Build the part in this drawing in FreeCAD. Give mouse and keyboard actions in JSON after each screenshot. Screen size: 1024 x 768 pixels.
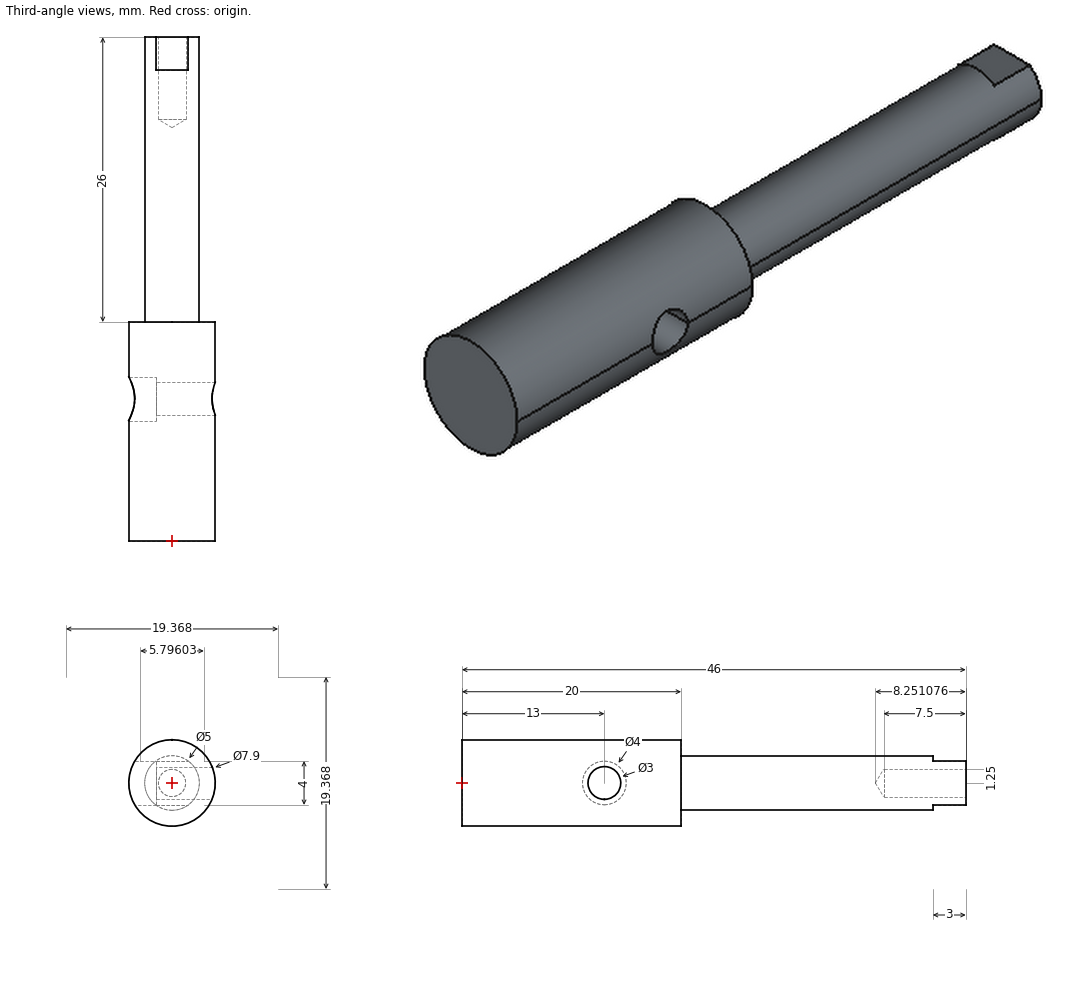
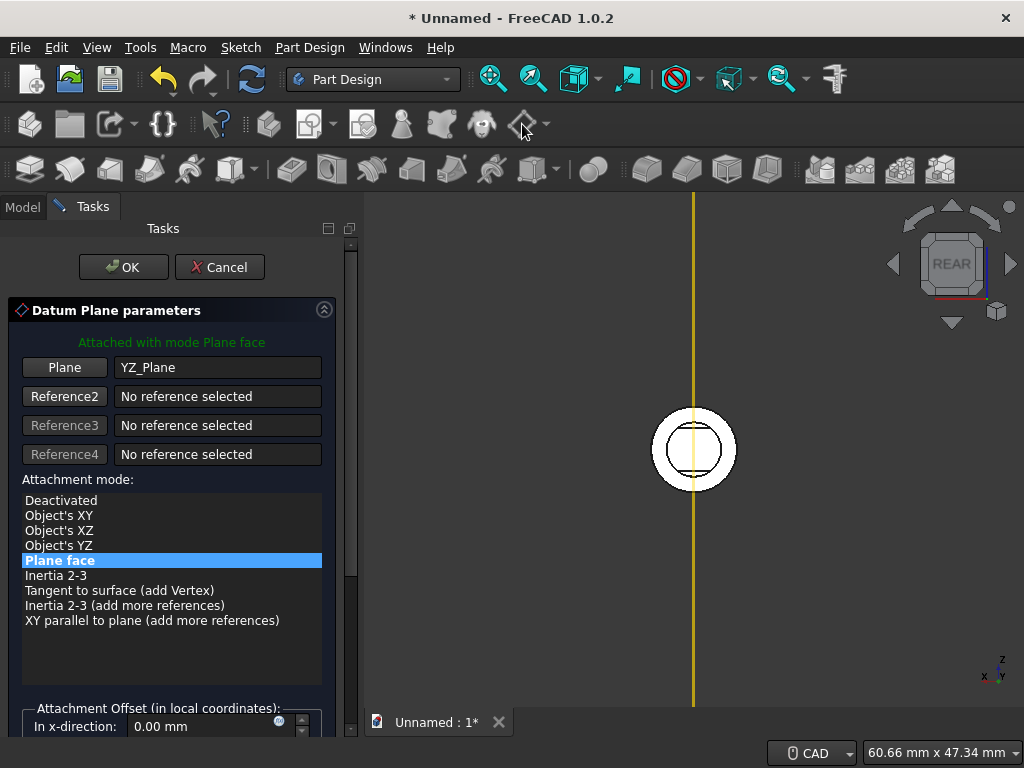
{"action": "scroll", "coordinate": [351, 487], "scroll_direction": "down", "scroll_amount": 3}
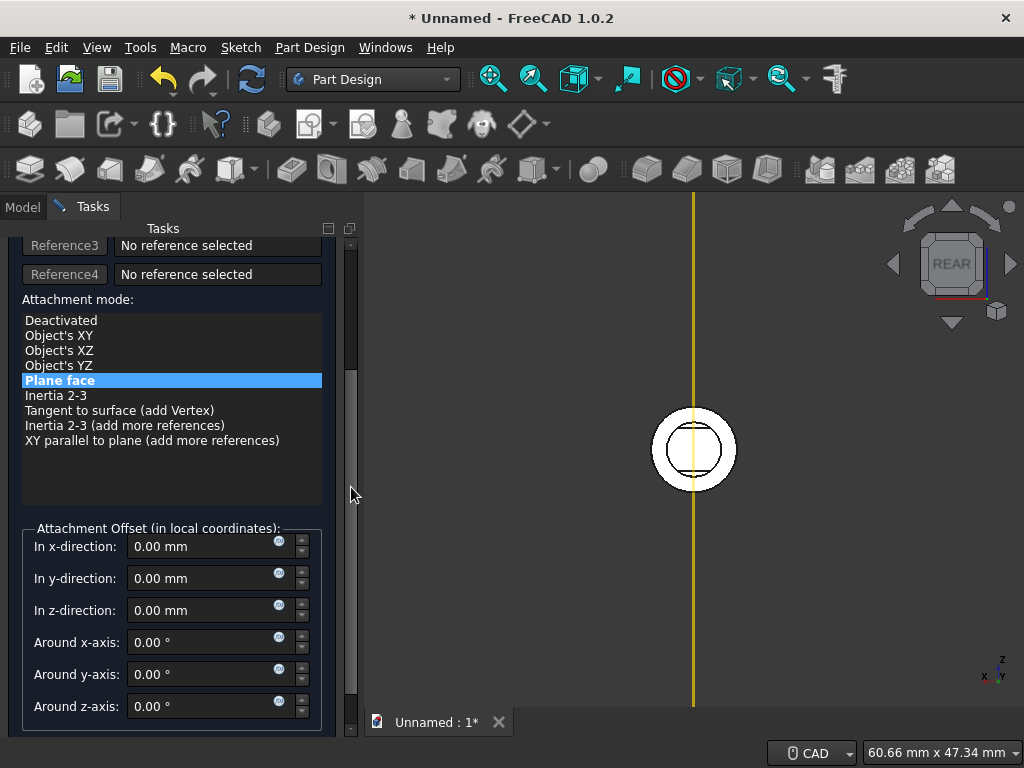
{"action": "triple_click", "coordinate": [210, 610]}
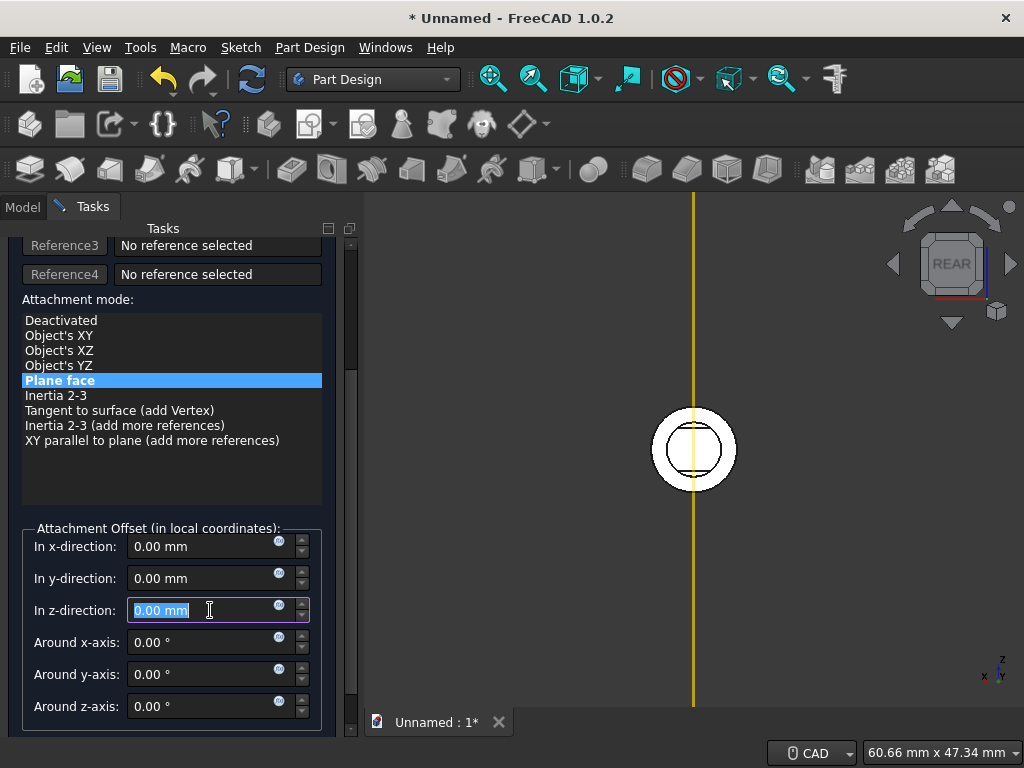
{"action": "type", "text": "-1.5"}
{"action": "key", "text": "Tab"}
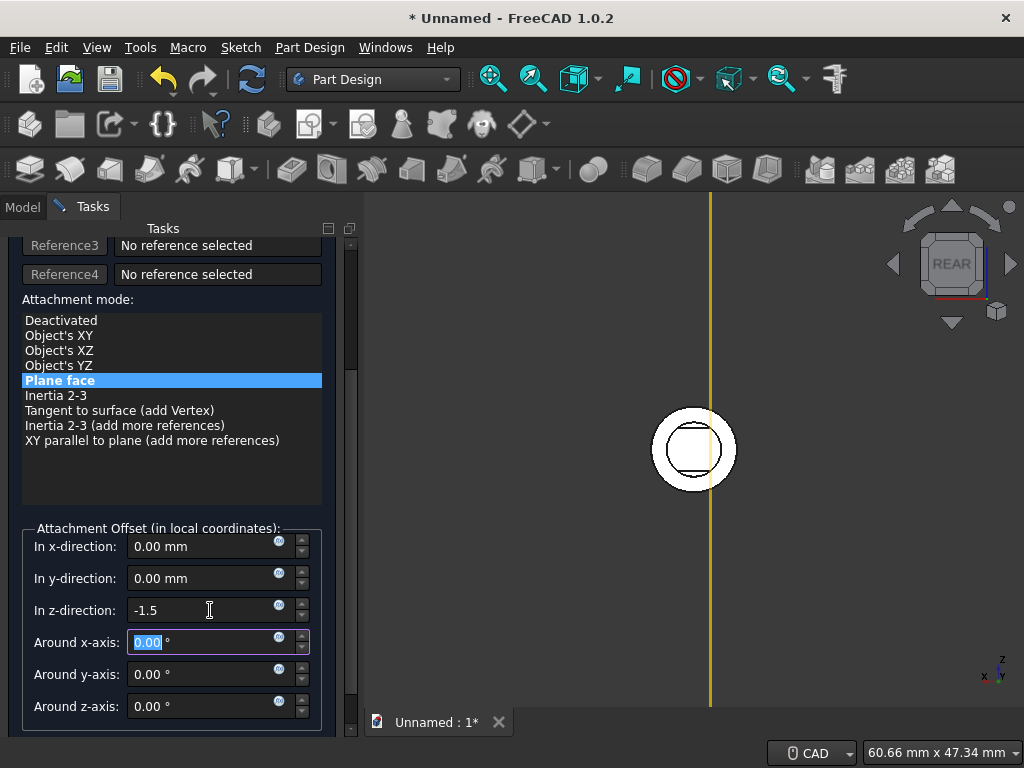
{"action": "scroll", "coordinate": [351, 487], "scroll_direction": "up", "scroll_amount": 4}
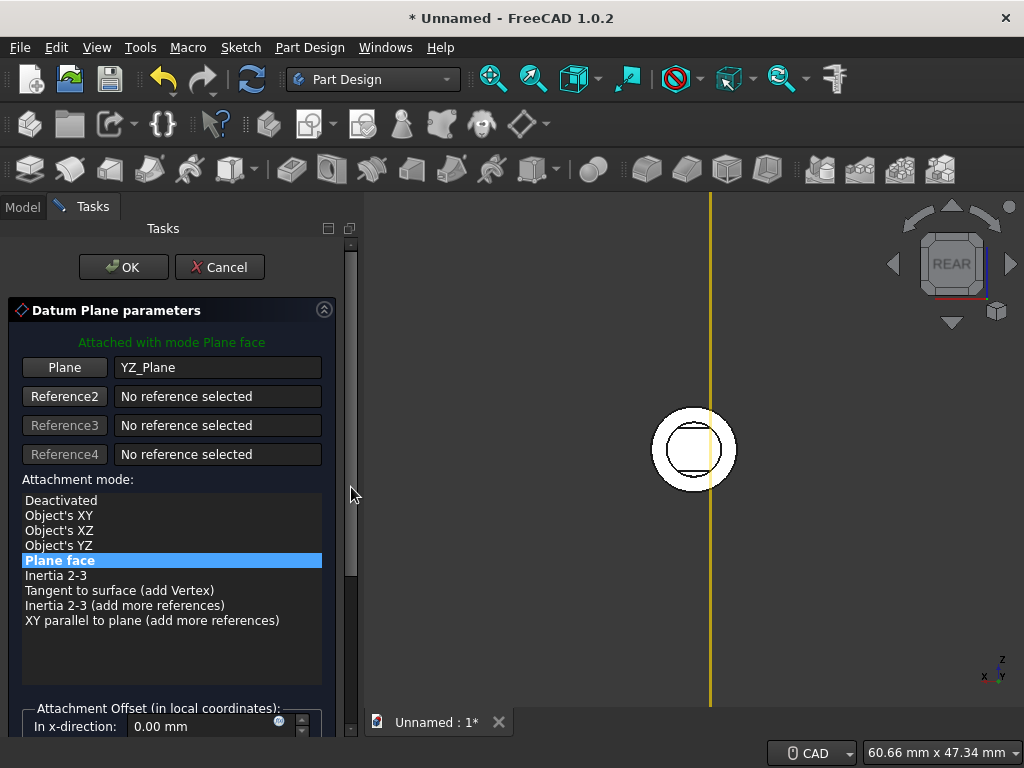
{"action": "left_click", "coordinate": [124, 267]}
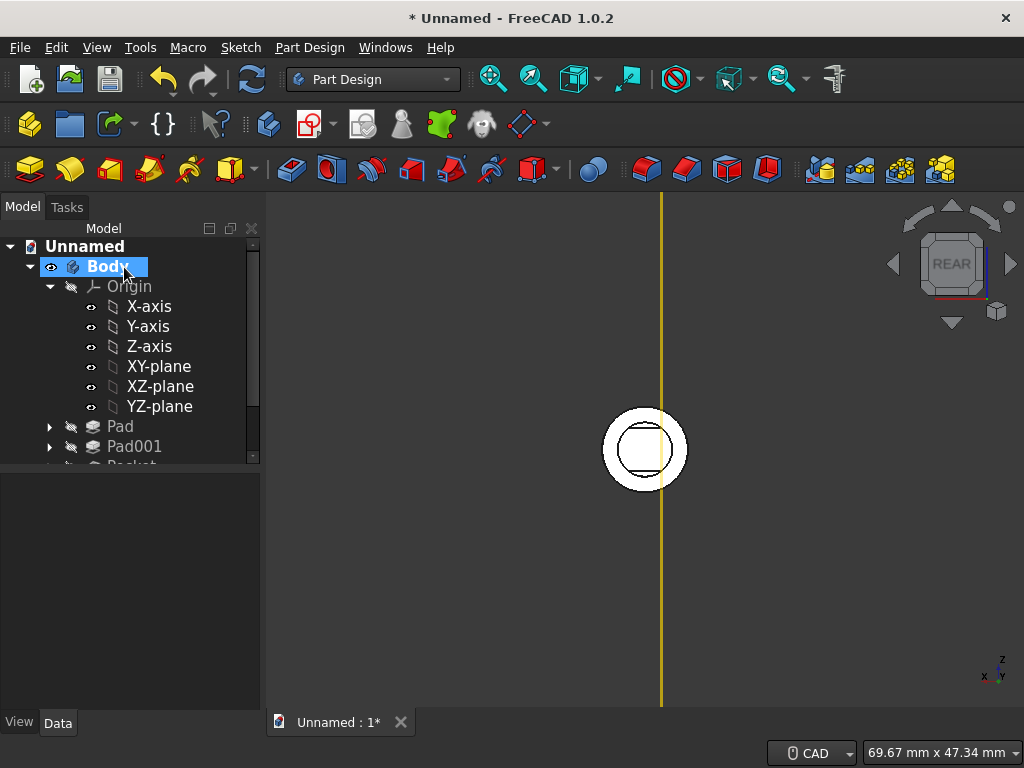
{"action": "scroll", "coordinate": [100, 342], "scroll_direction": "down", "scroll_amount": 3}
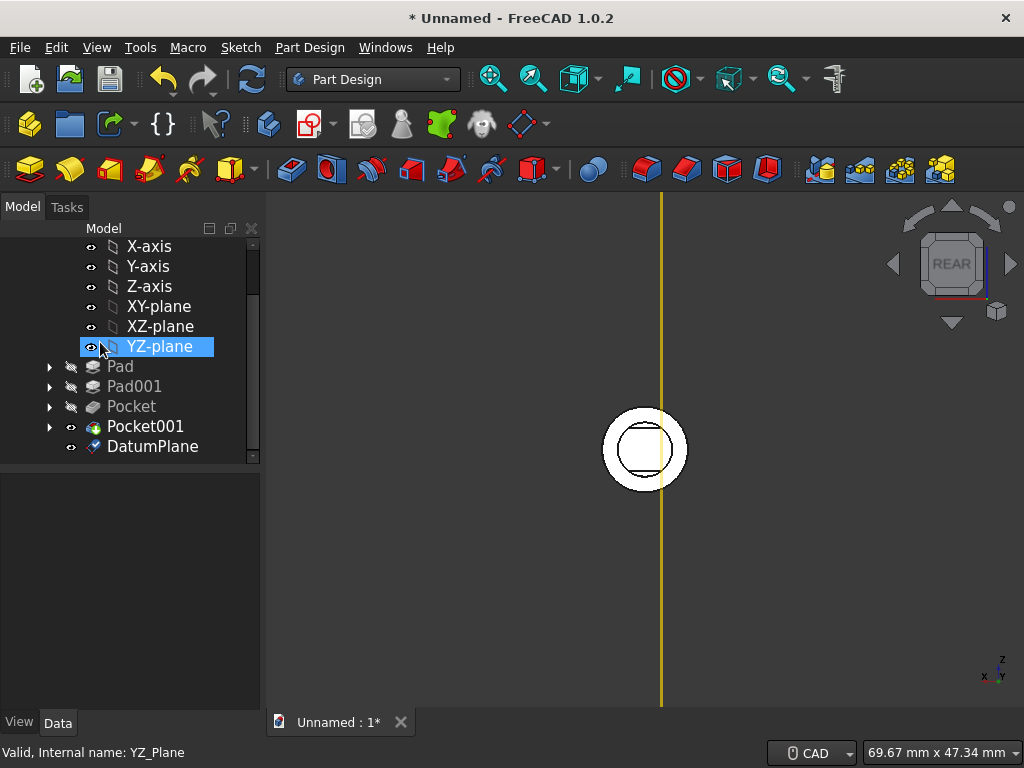
{"action": "left_click", "coordinate": [116, 447]}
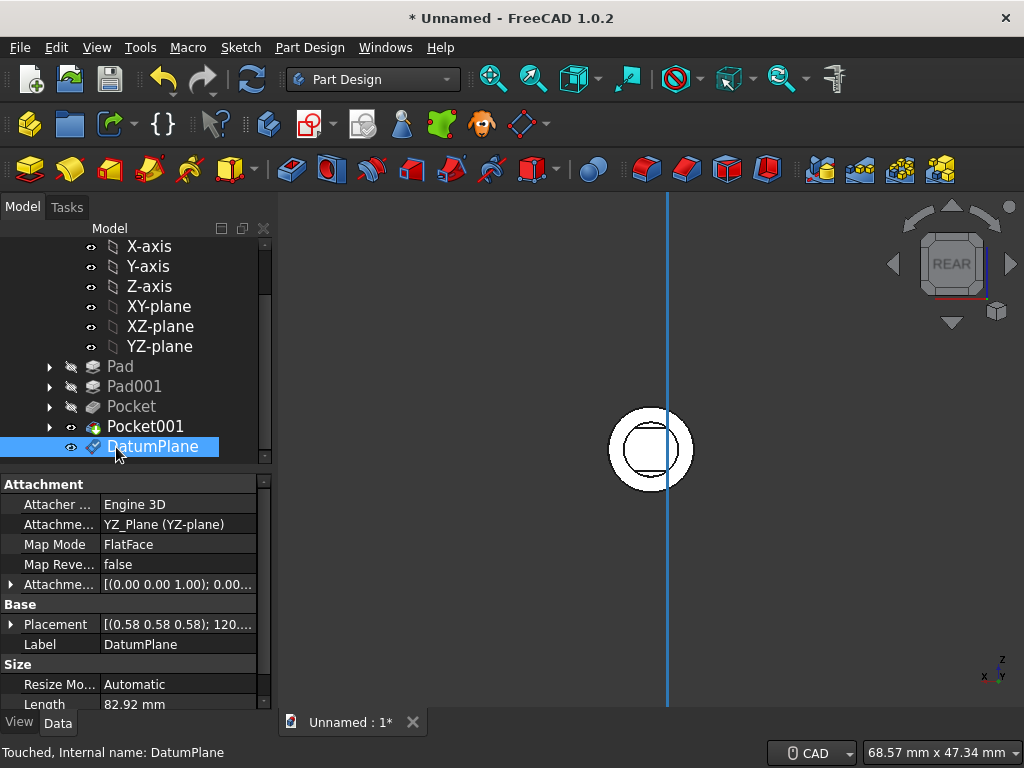
{"action": "left_click", "coordinate": [310, 124]}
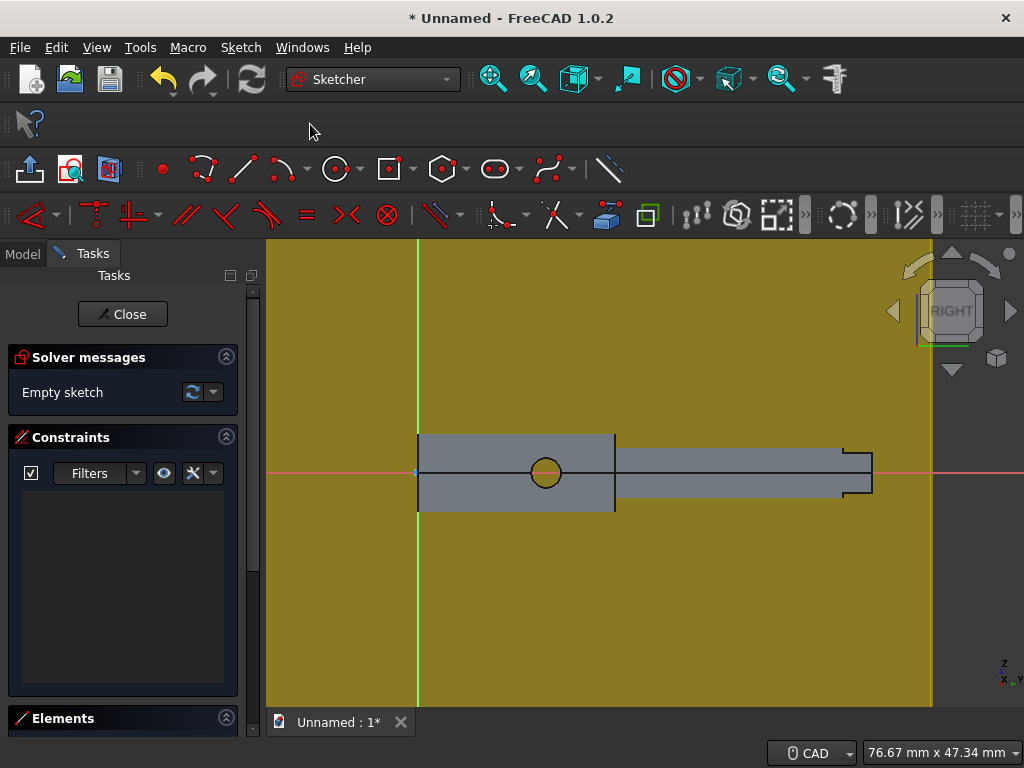
{"action": "left_click", "coordinate": [110, 170]}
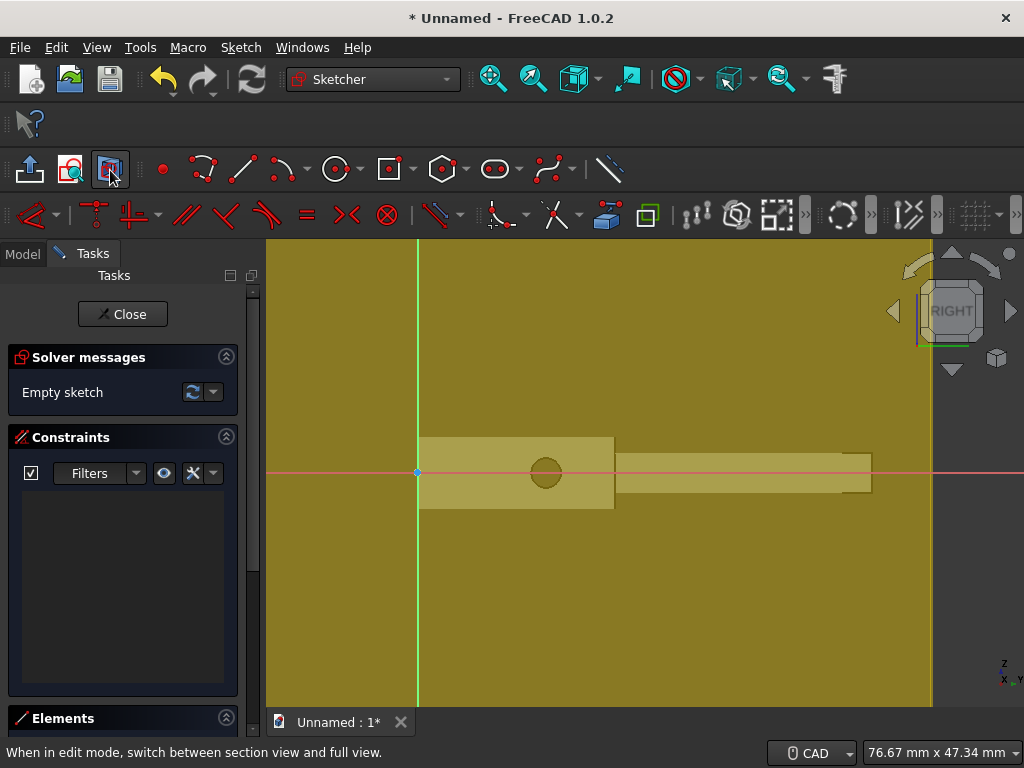
{"action": "scroll", "coordinate": [541, 473], "scroll_direction": "up", "scroll_amount": 10}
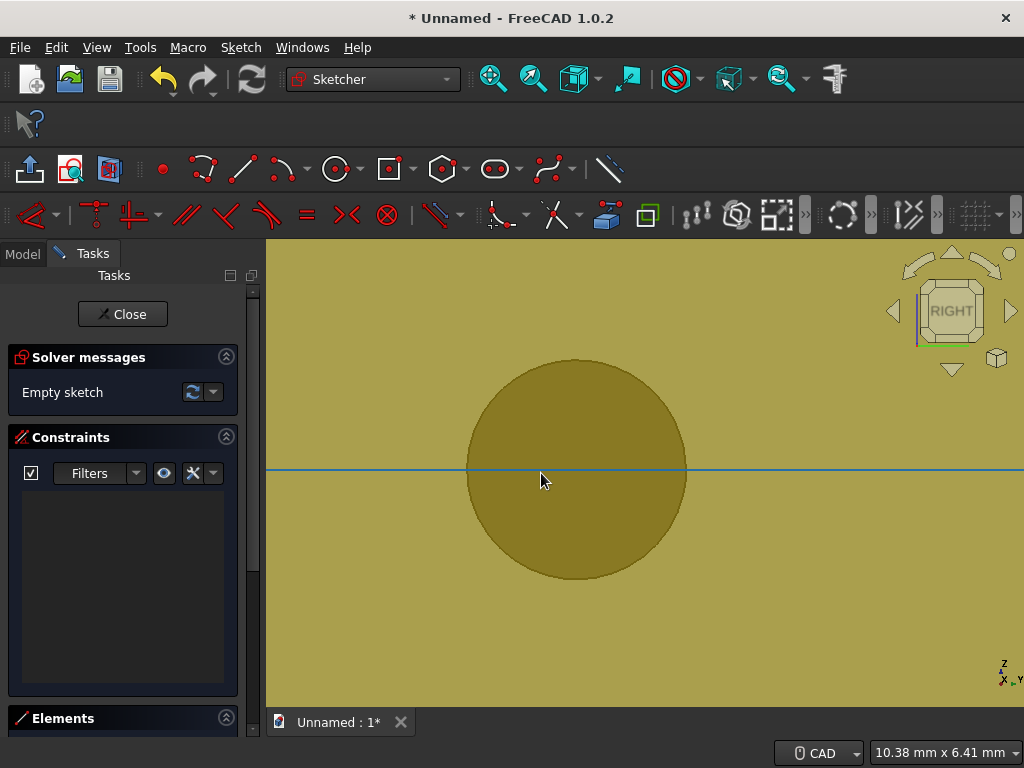
{"action": "left_click", "coordinate": [336, 170]}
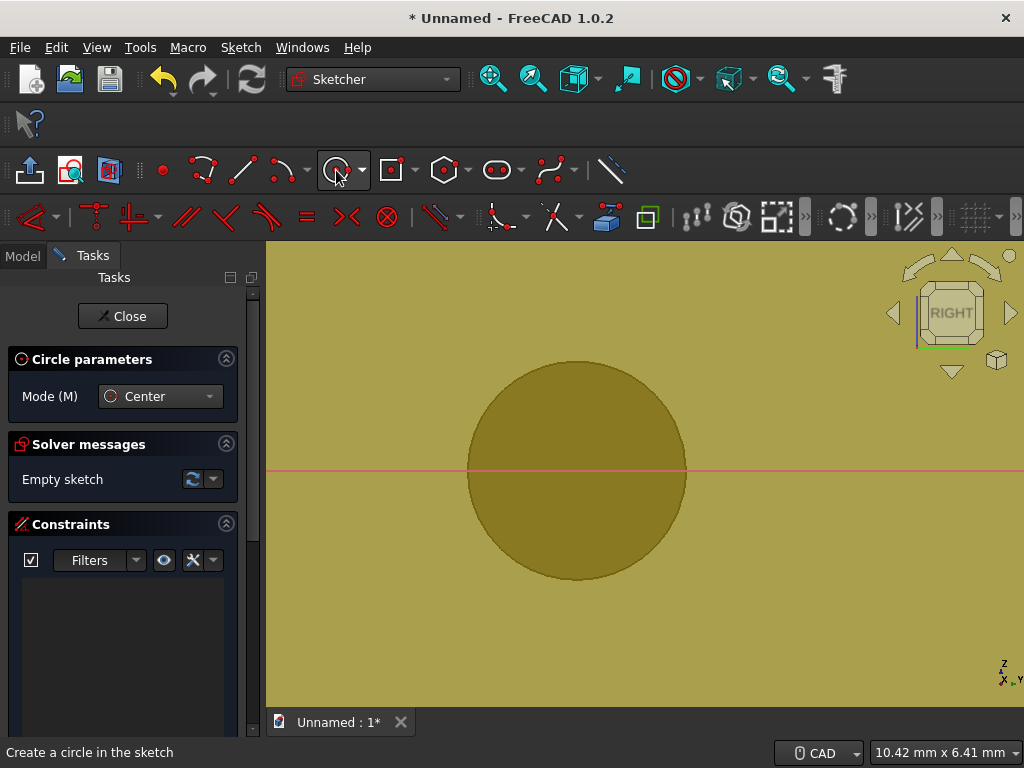
{"action": "left_click", "coordinate": [577, 471]}
{"action": "mouse_move", "coordinate": [680, 368]}